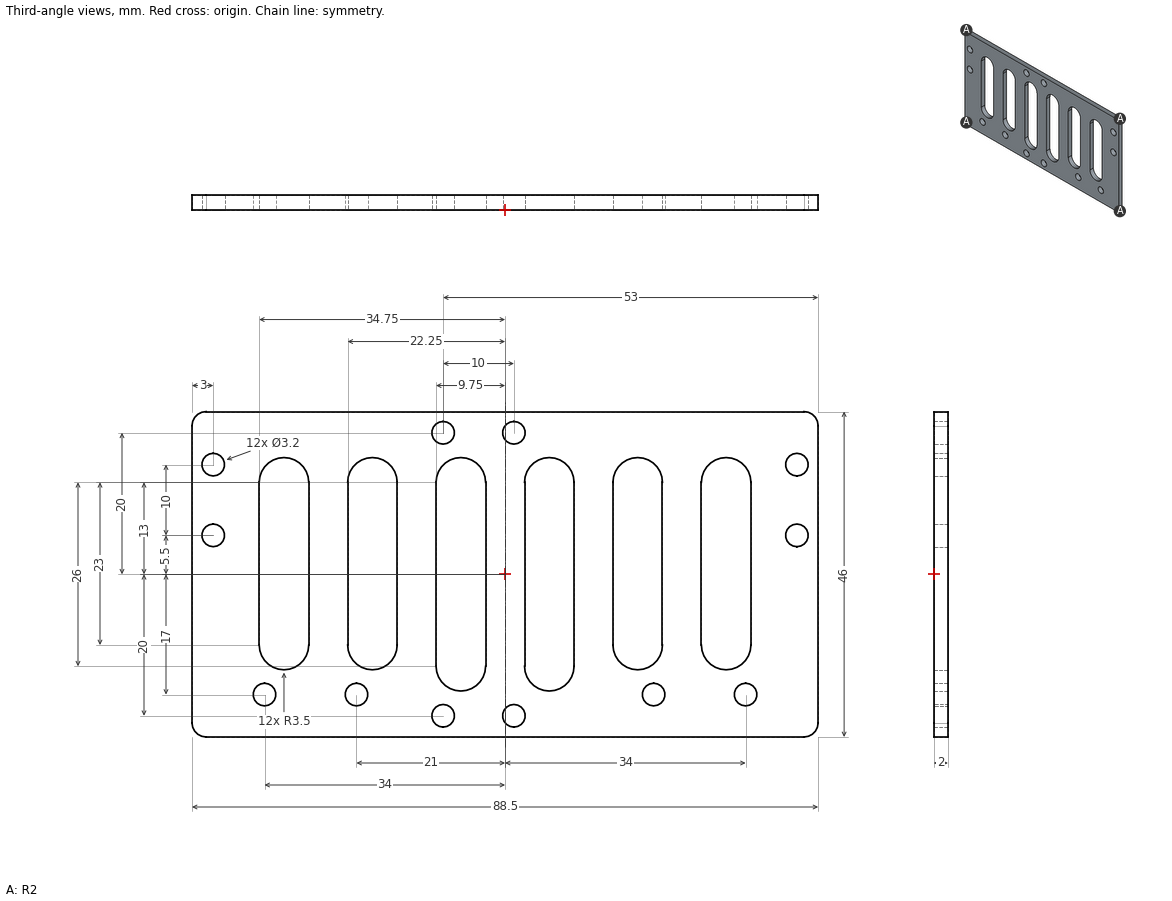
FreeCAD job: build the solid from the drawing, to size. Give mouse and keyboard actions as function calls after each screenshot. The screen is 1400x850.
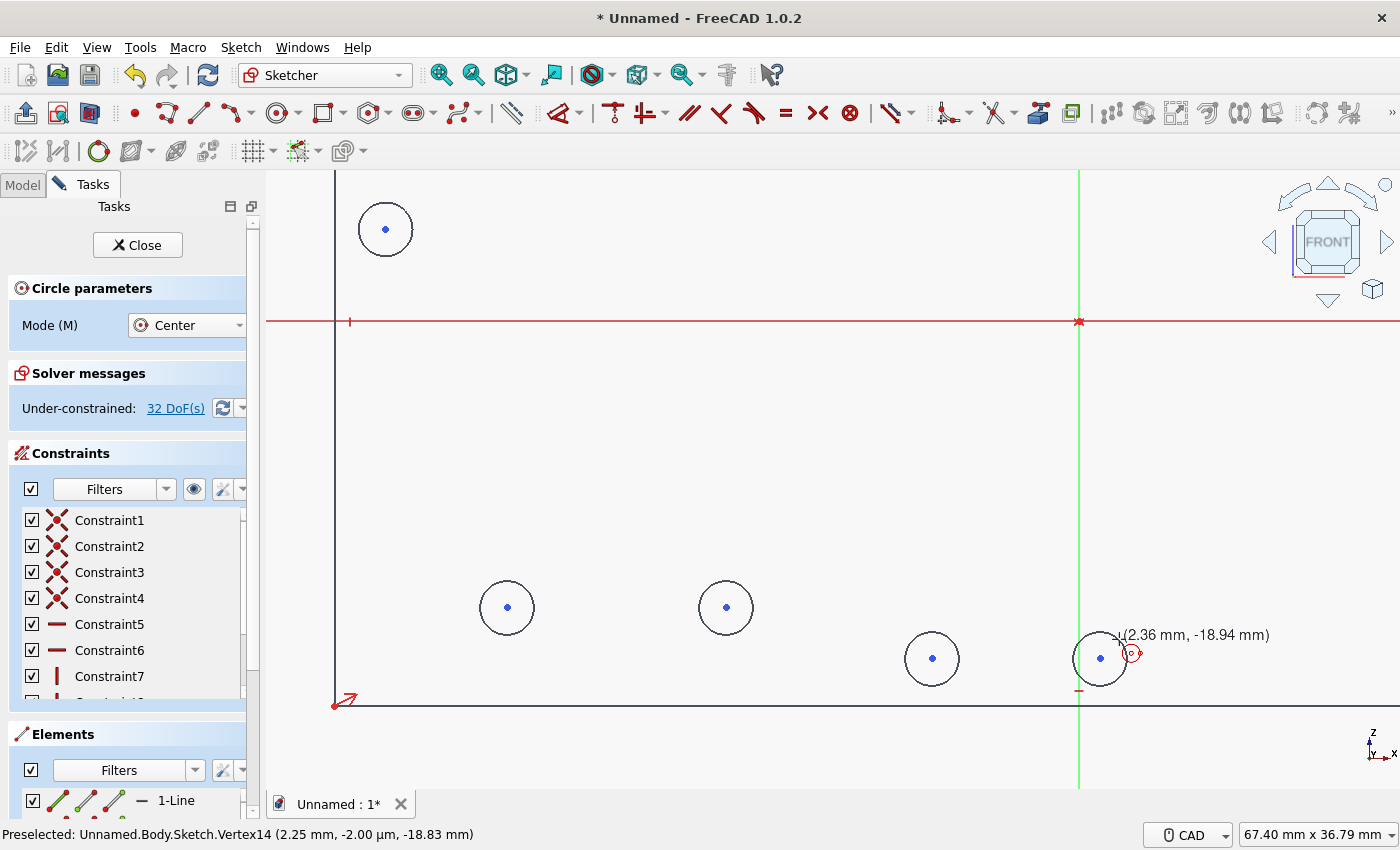
scroll(508, 609, down, 4)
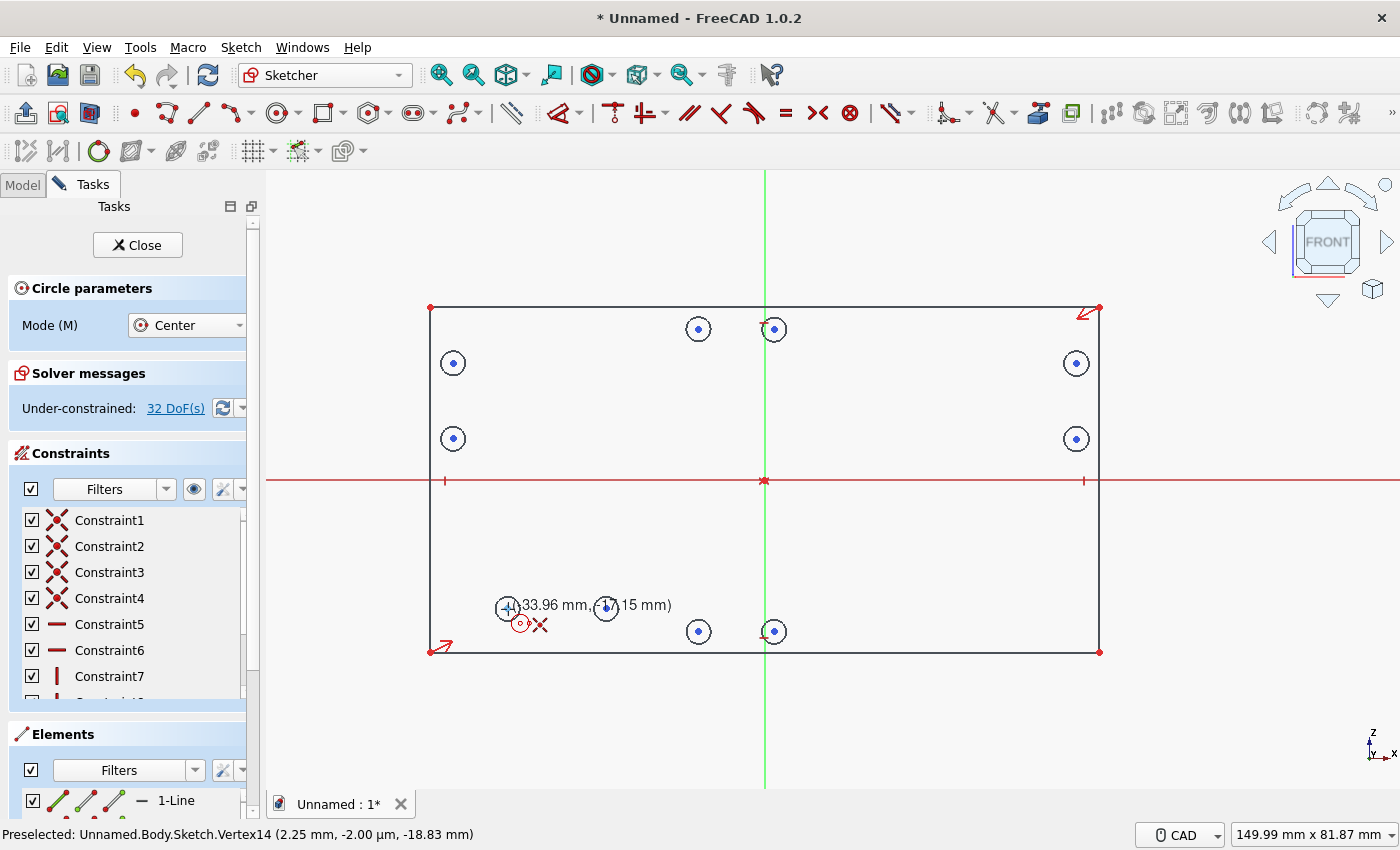
scroll(924, 609, up, 4)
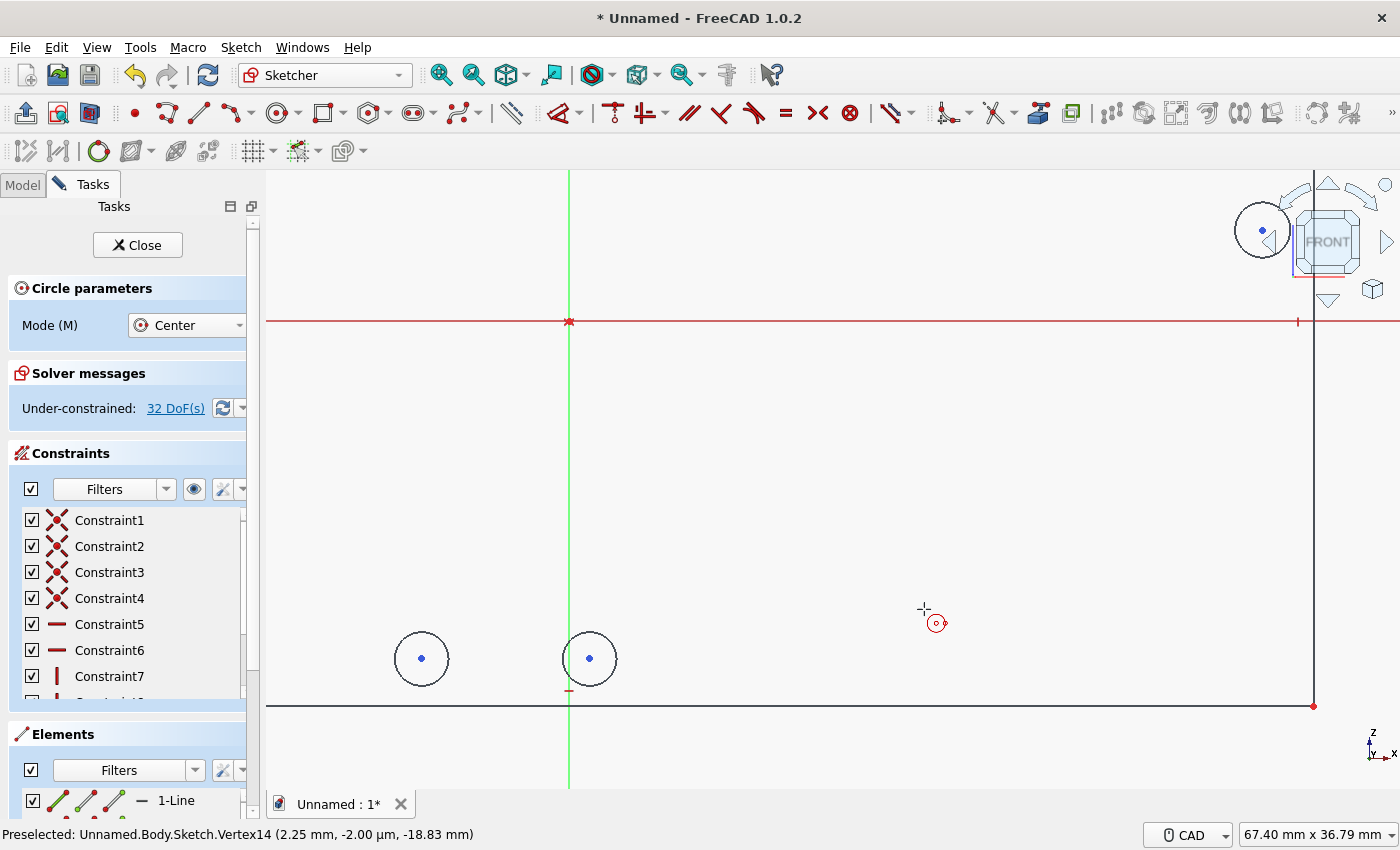
click(922, 607)
click(941, 588)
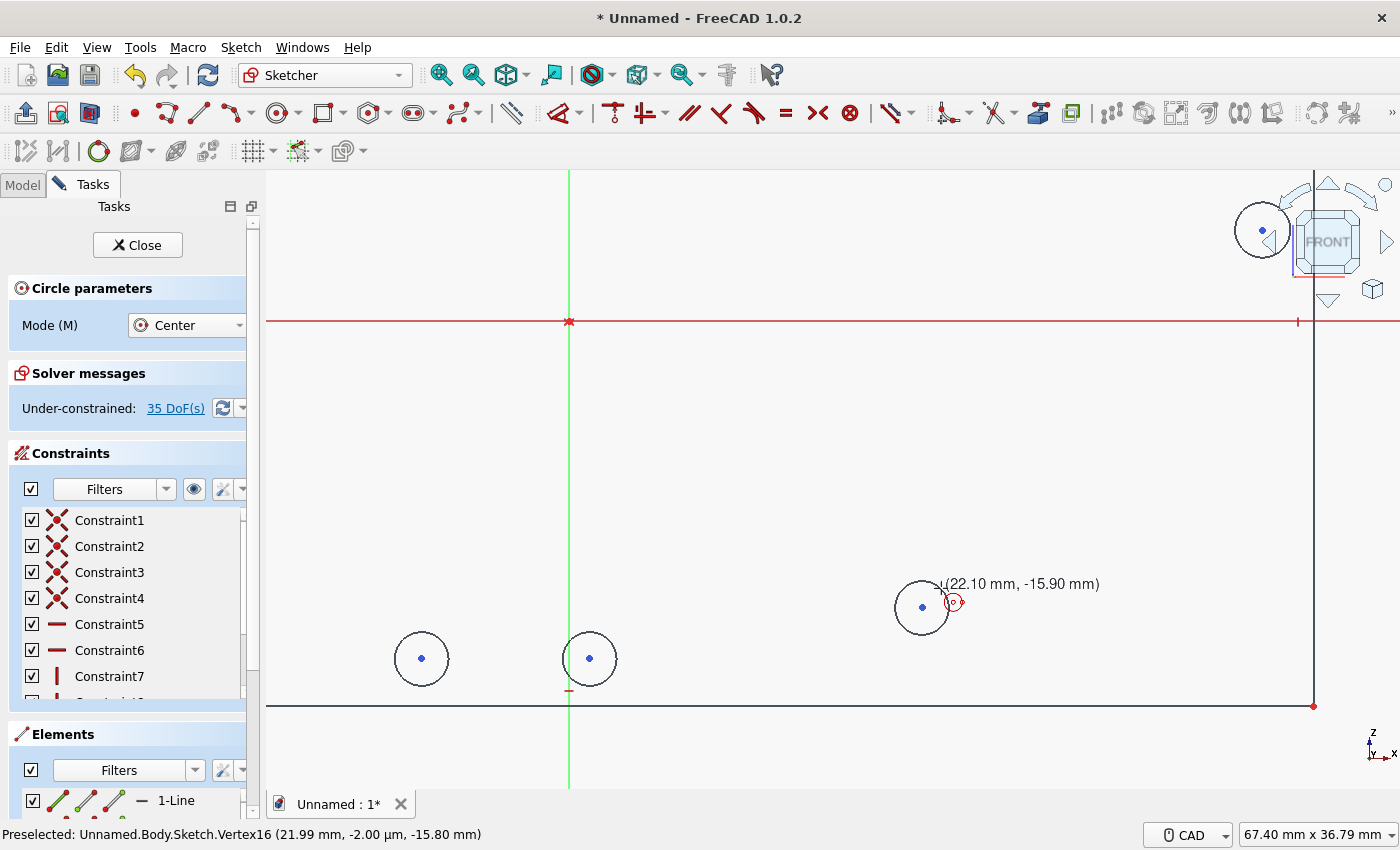
click(1141, 607)
click(1160, 588)
key(Escape)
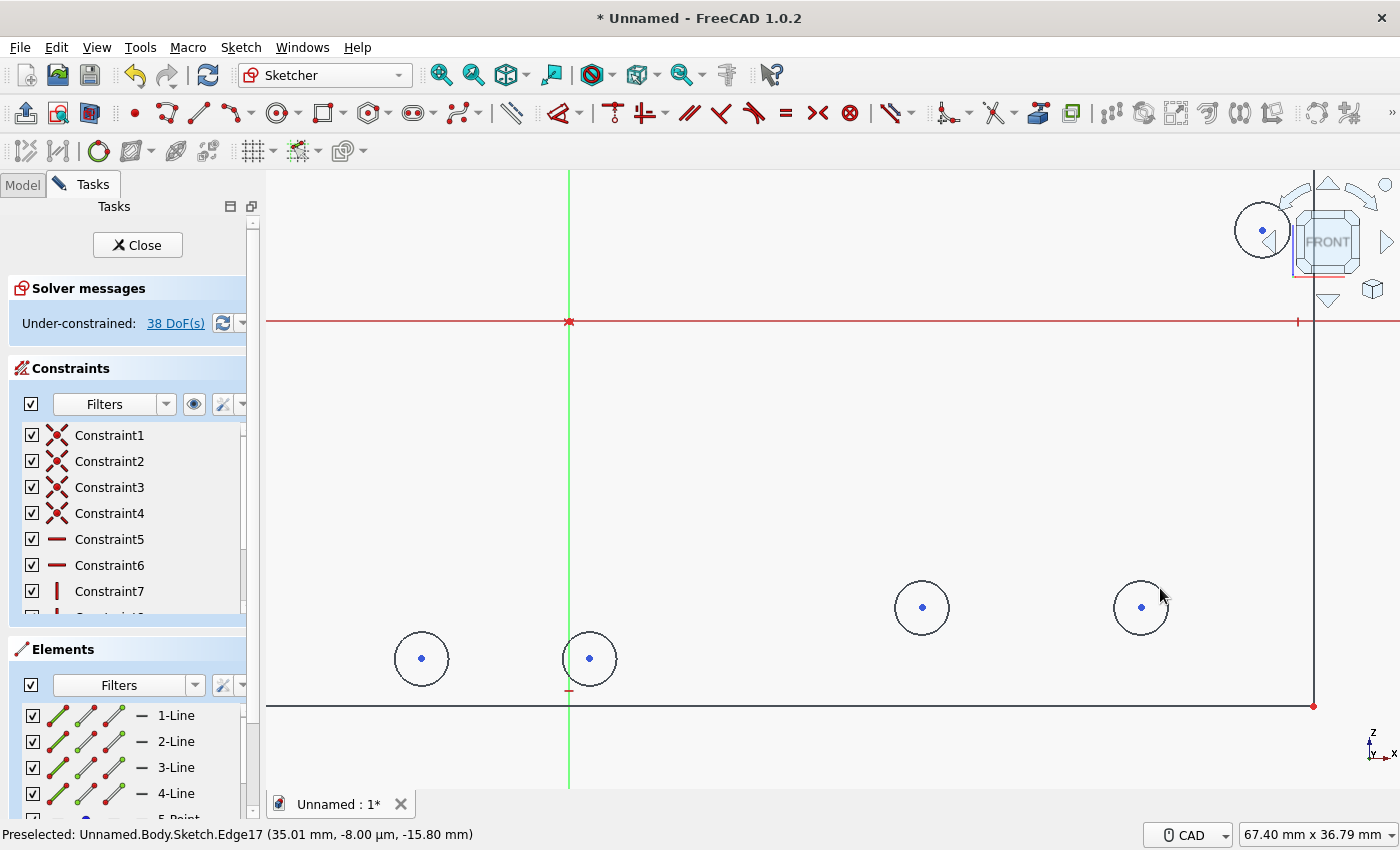
scroll(924, 609, down, 4)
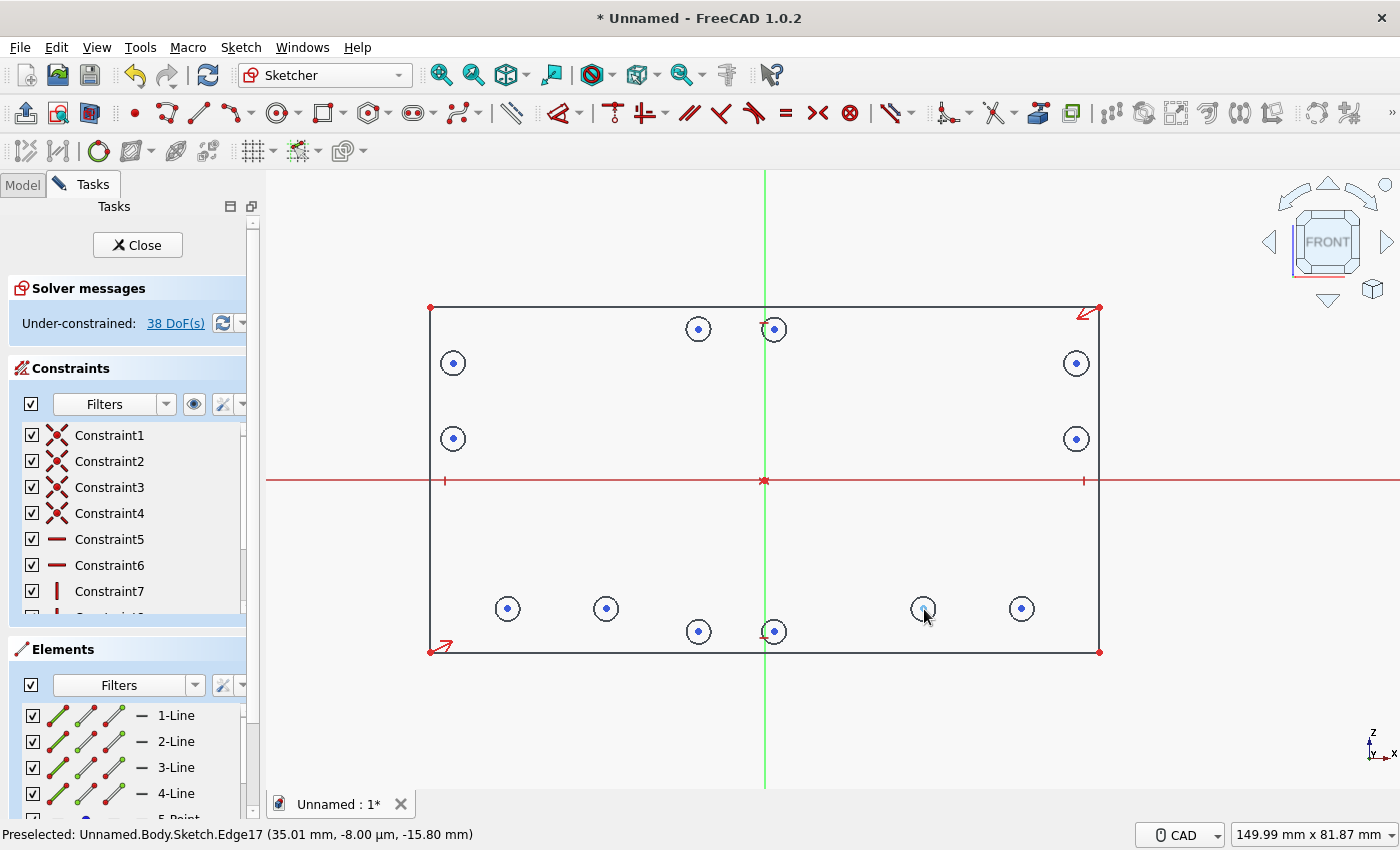
click(462, 355)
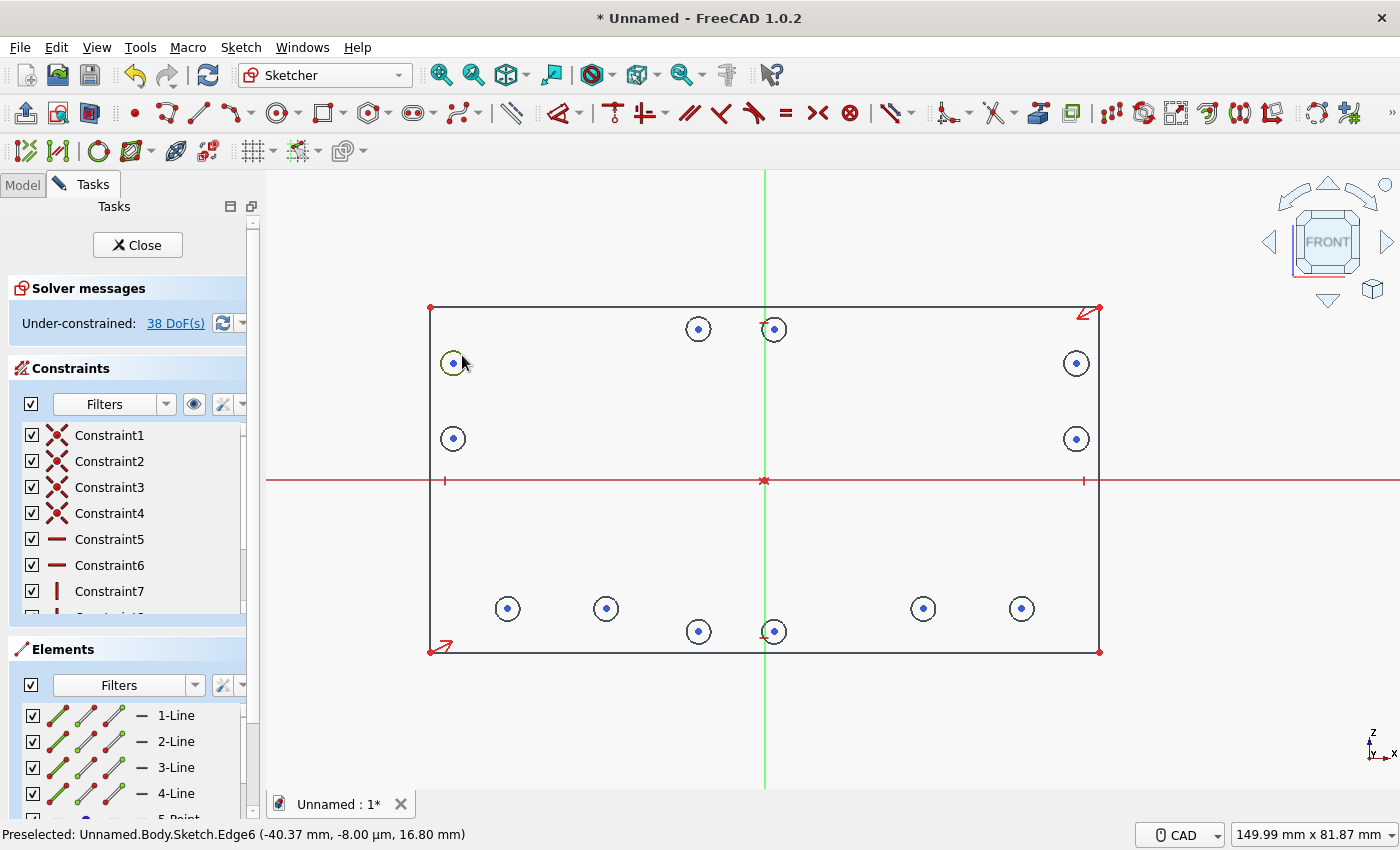
click(707, 321)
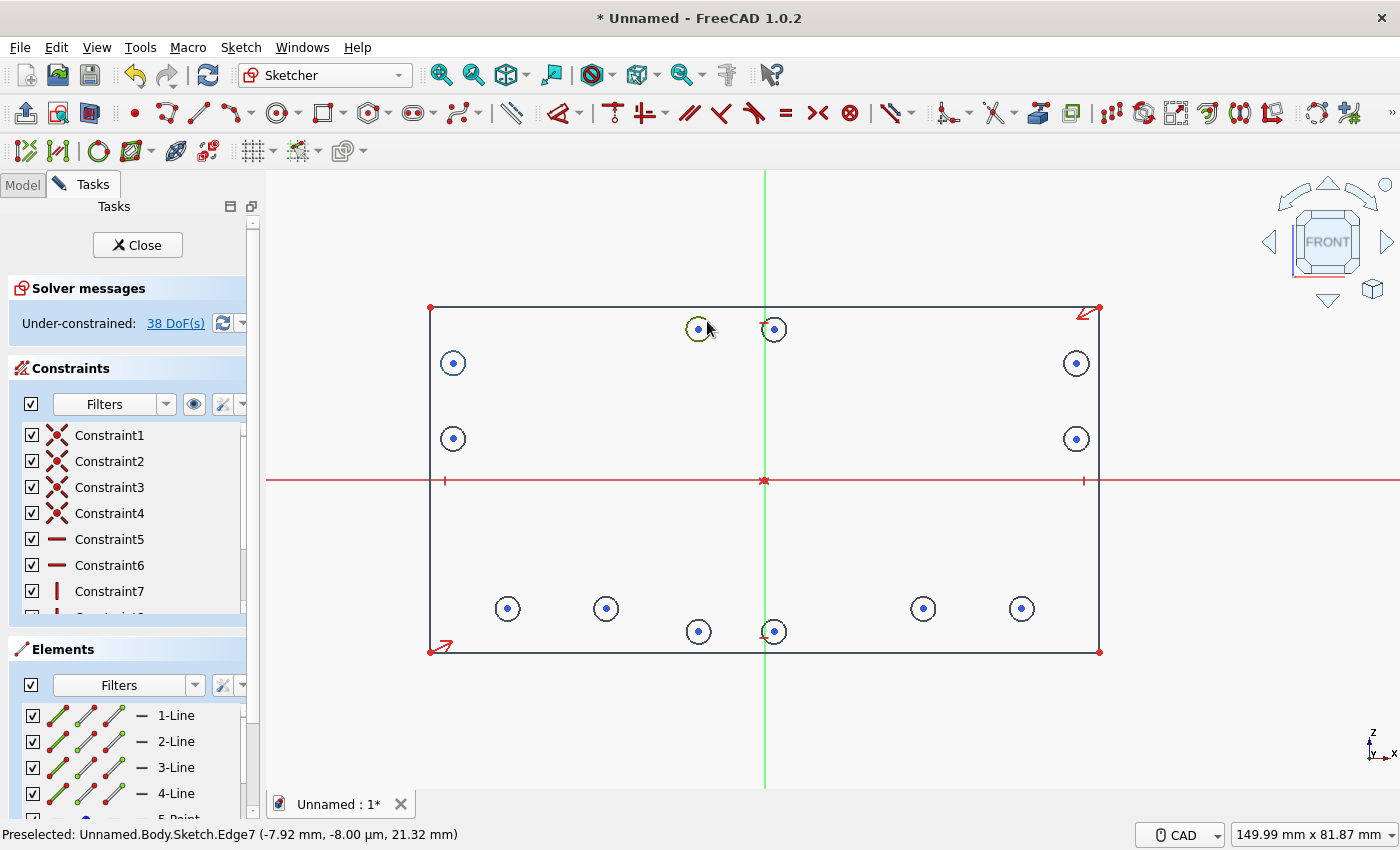
click(462, 430)